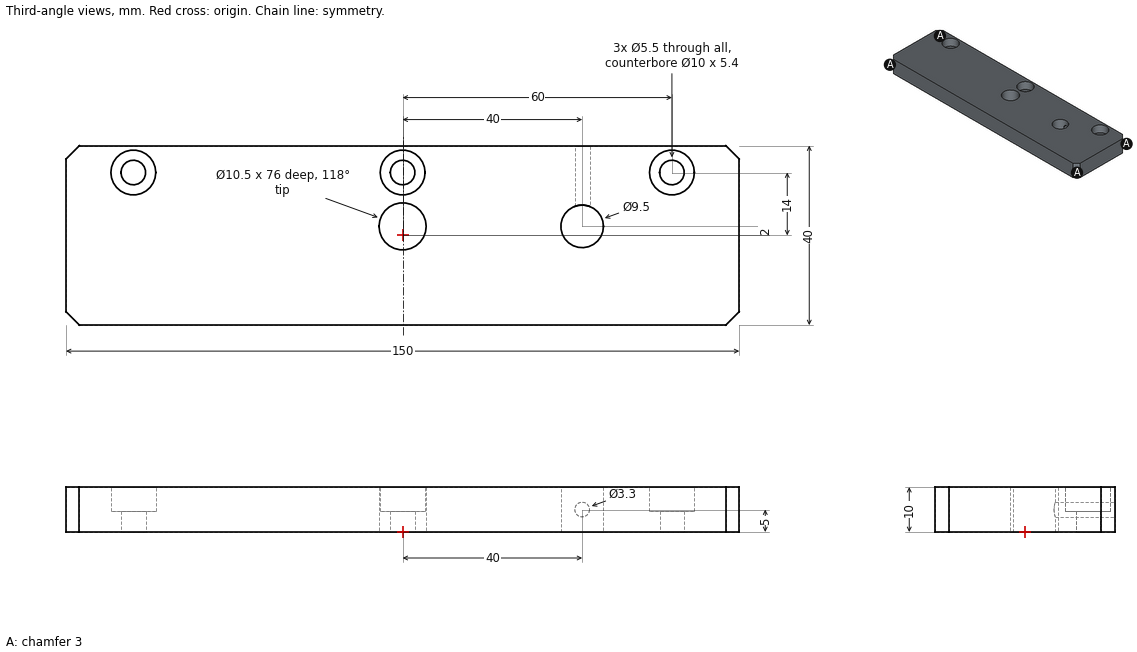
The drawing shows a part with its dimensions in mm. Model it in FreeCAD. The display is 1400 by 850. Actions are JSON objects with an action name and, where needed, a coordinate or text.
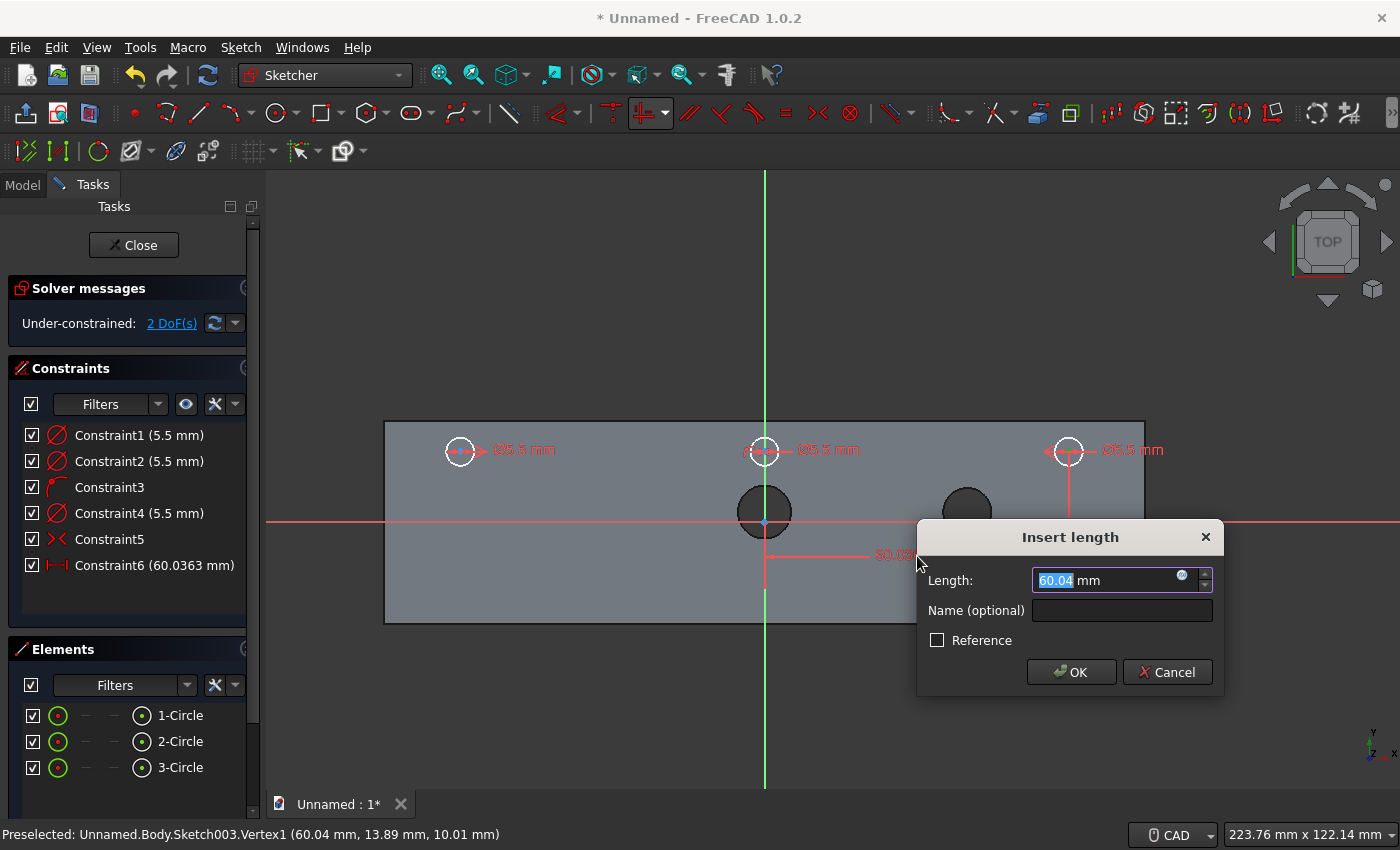
{"action": "type", "text": "60"}
{"action": "key", "text": "Return"}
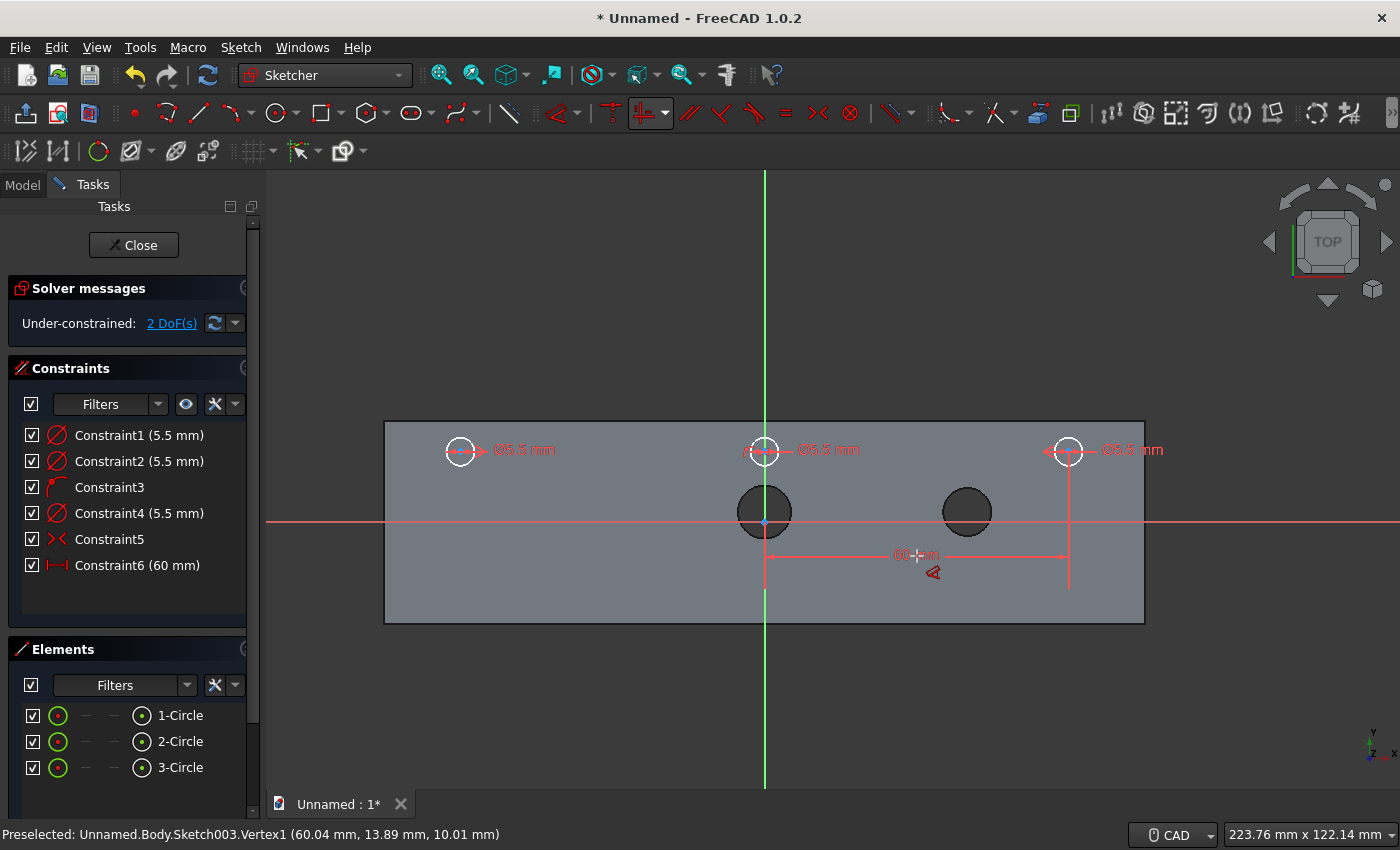
{"action": "left_click", "coordinate": [1069, 452]}
{"action": "left_click", "coordinate": [1103, 487]}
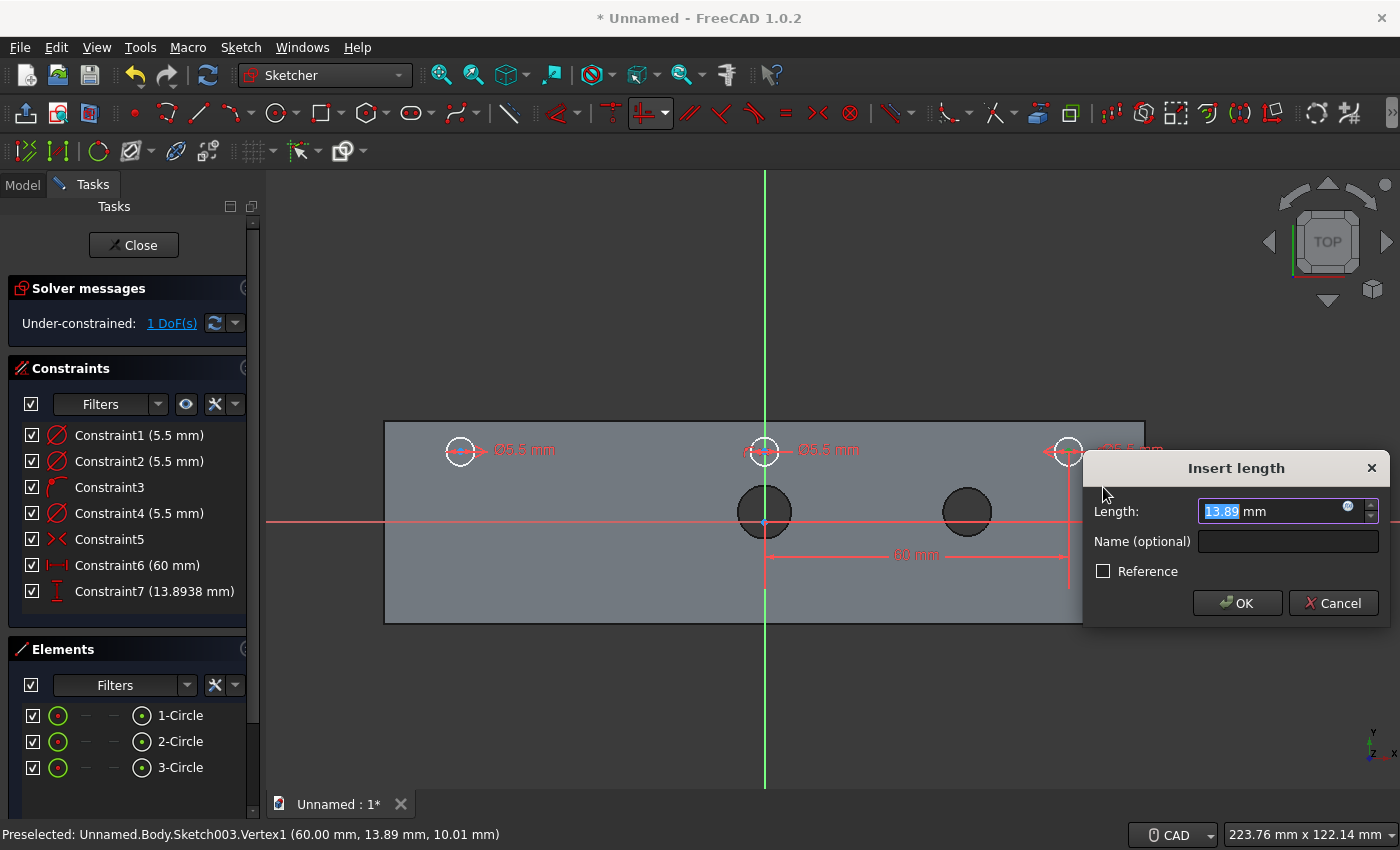
{"action": "type", "text": "14"}
{"action": "key", "text": "Return"}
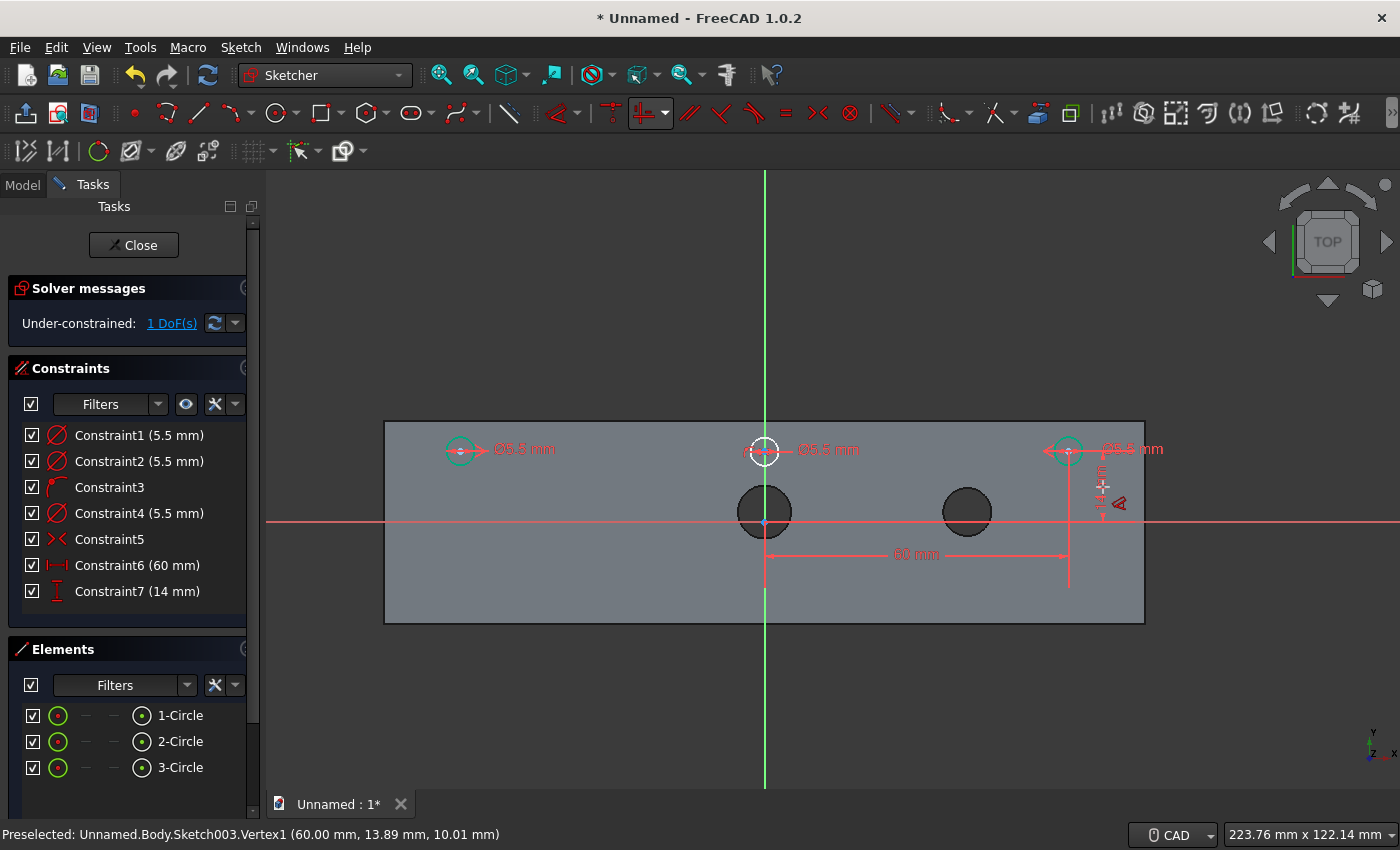
{"action": "left_click", "coordinate": [765, 452]}
{"action": "left_click", "coordinate": [799, 487]}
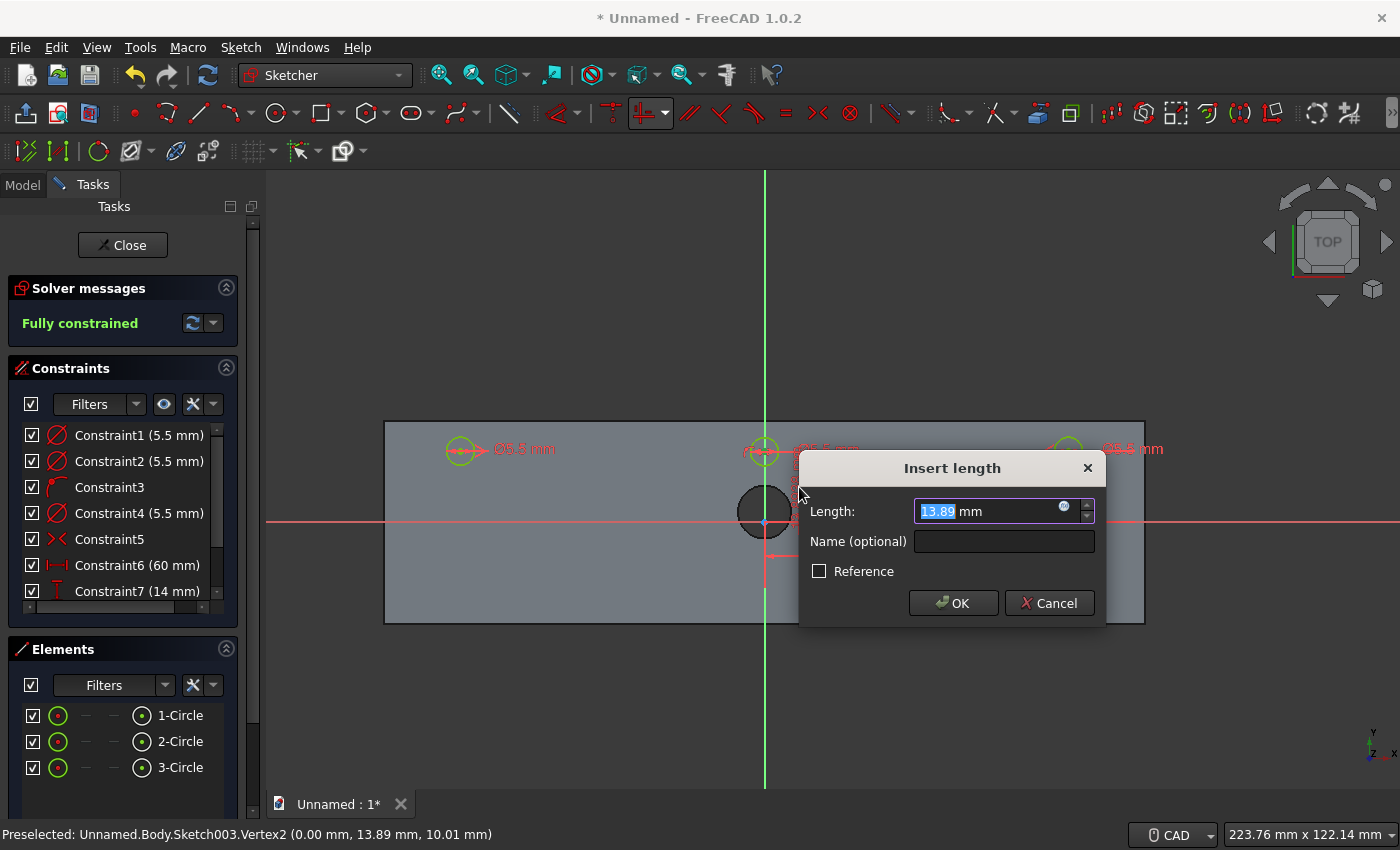
{"action": "type", "text": "14"}
{"action": "key", "text": "Return"}
{"action": "key", "text": "Escape"}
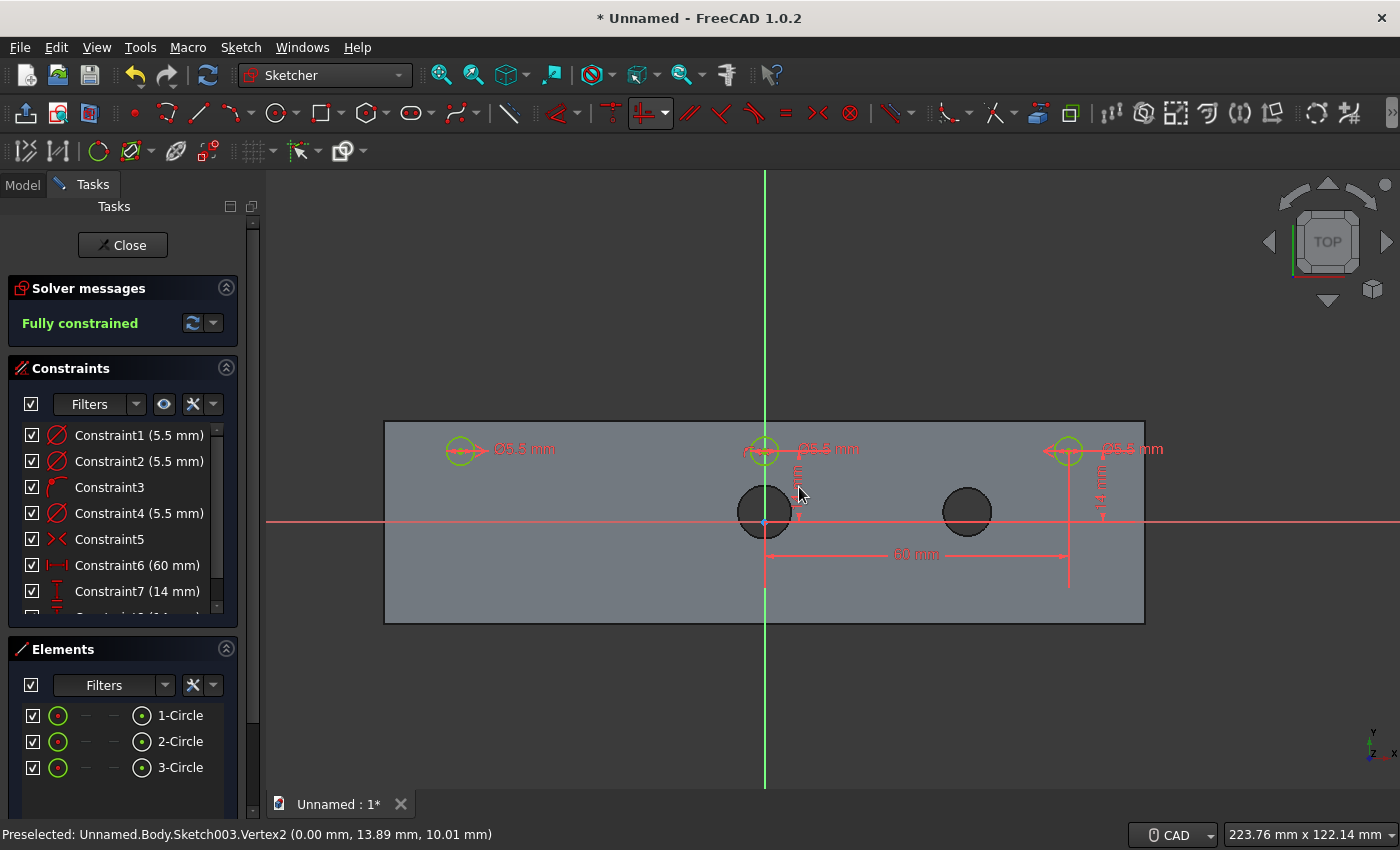
{"action": "left_click", "coordinate": [123, 245]}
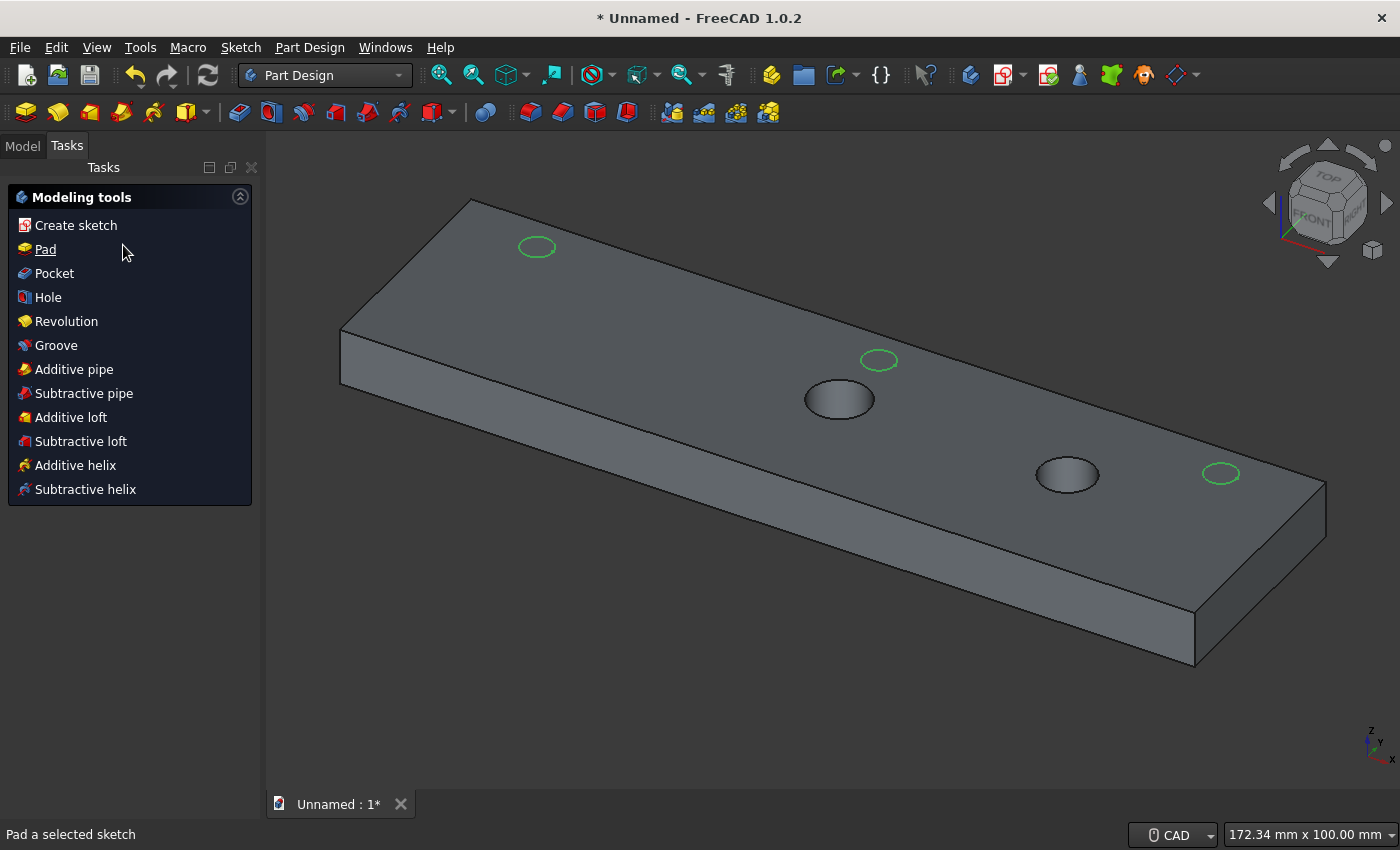
{"action": "left_click", "coordinate": [272, 112]}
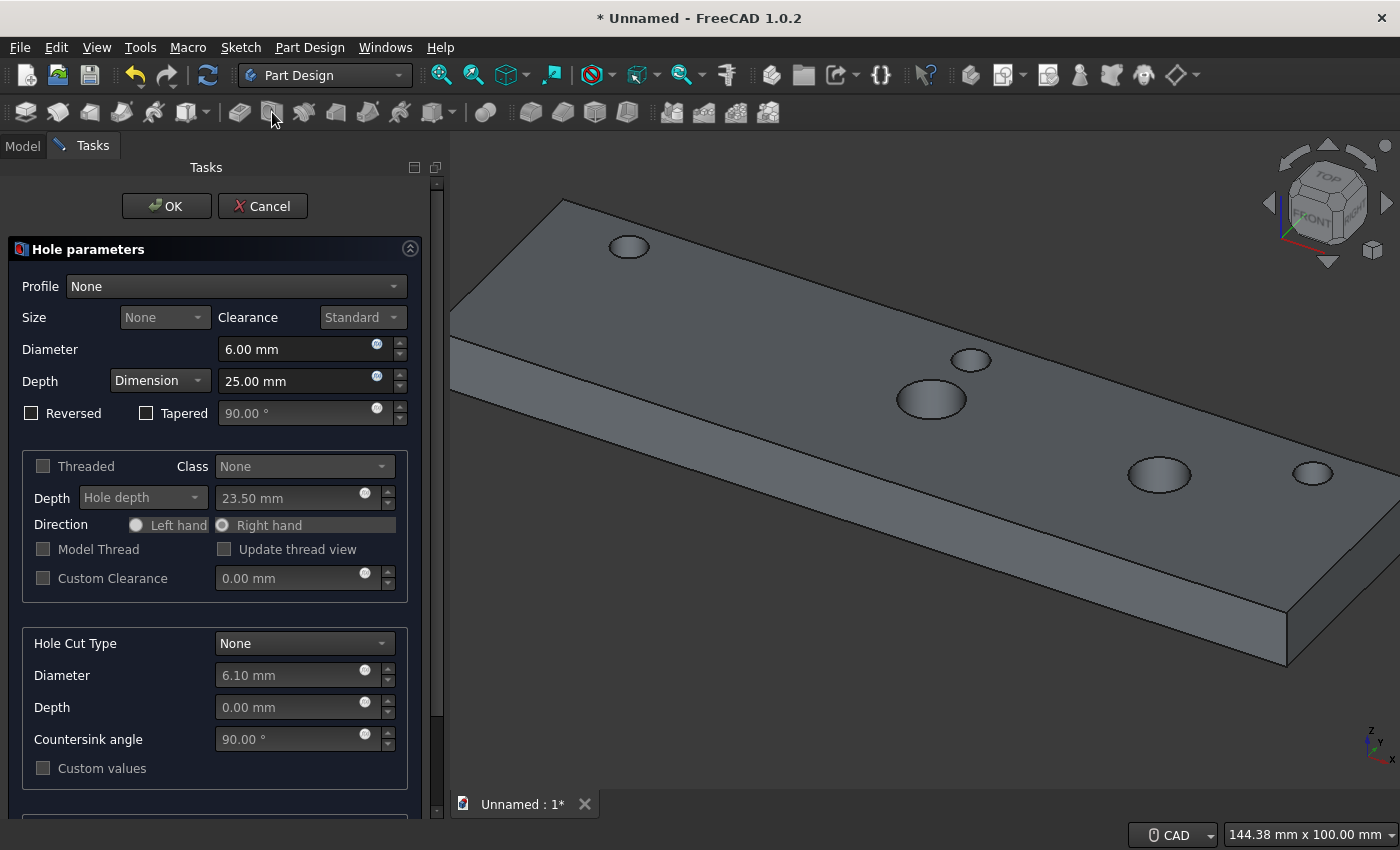
{"action": "triple_click", "coordinate": [305, 349]}